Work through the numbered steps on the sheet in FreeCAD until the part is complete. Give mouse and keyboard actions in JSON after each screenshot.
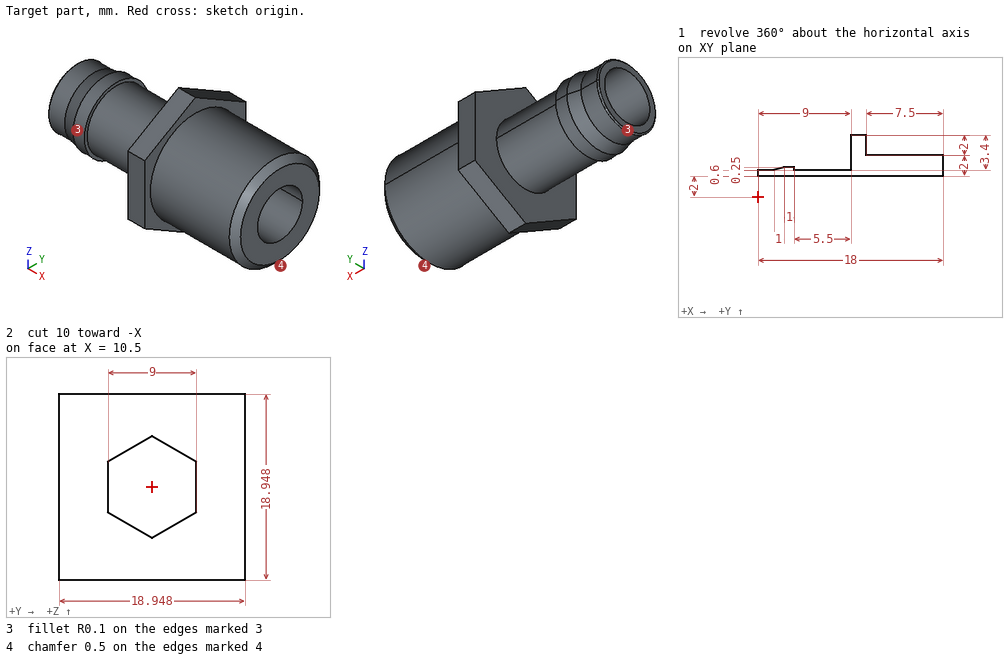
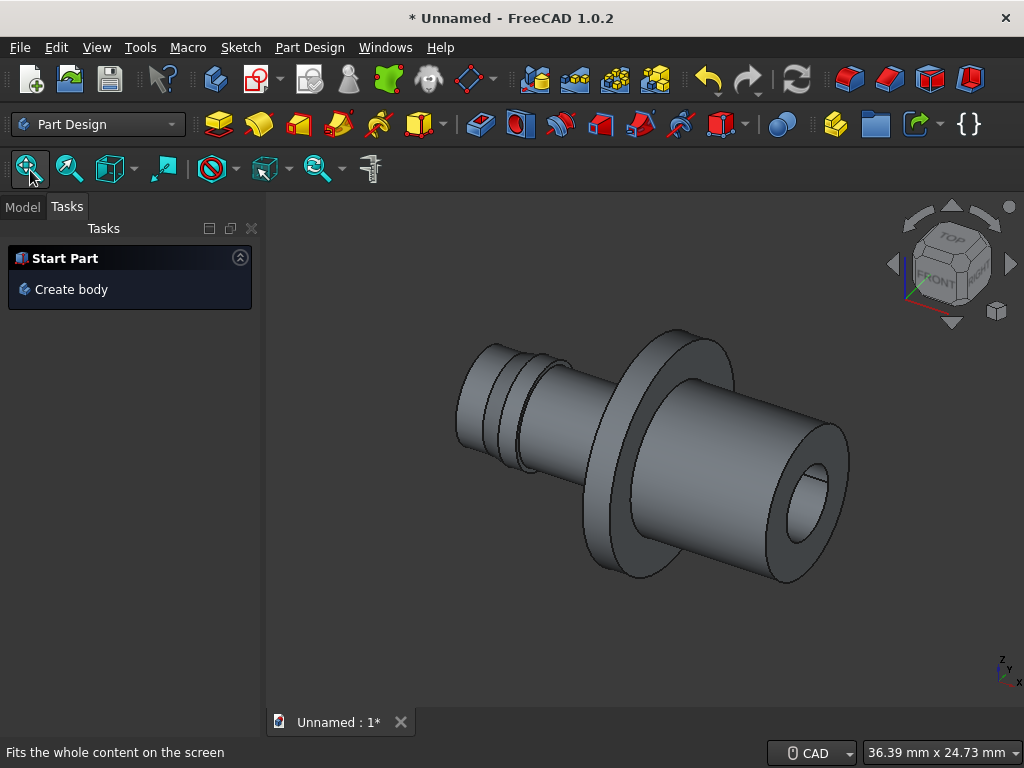
{"action": "left_click", "coordinate": [672, 370]}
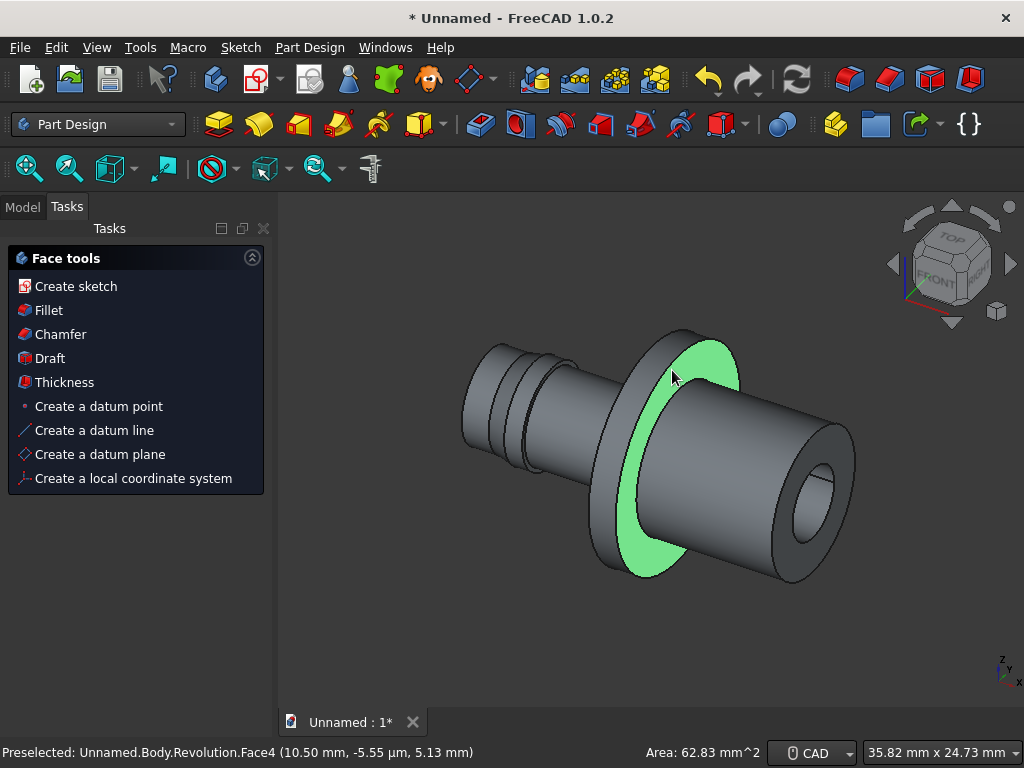
{"action": "left_click", "coordinate": [256, 80]}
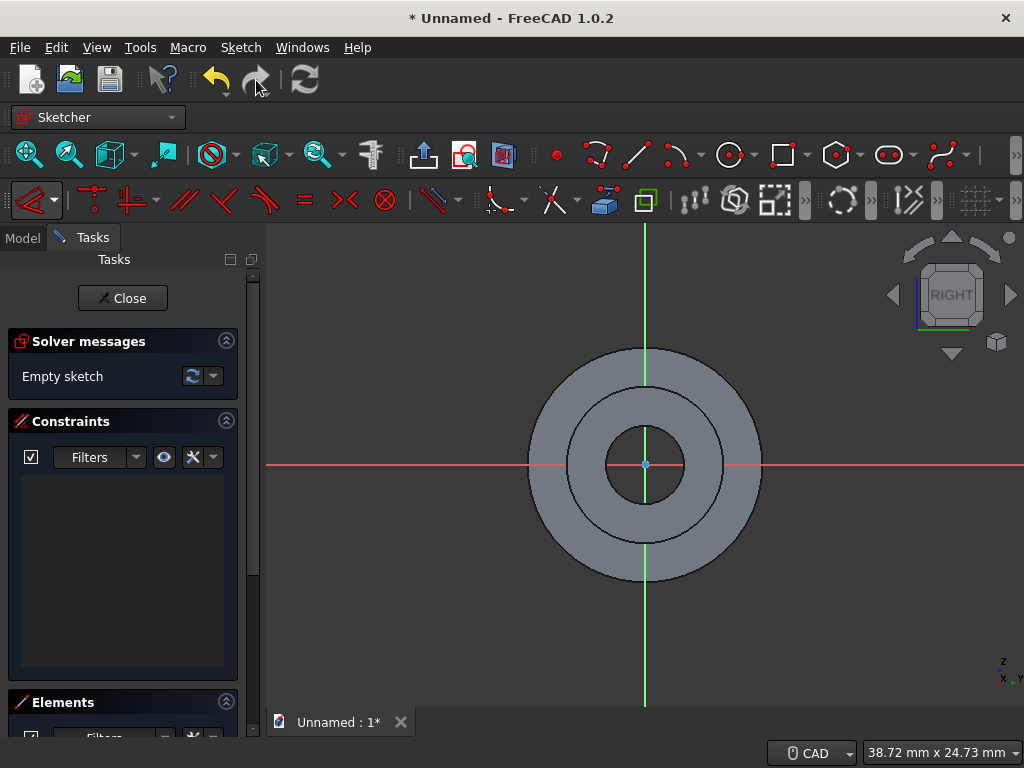
{"action": "left_click", "coordinate": [504, 156]}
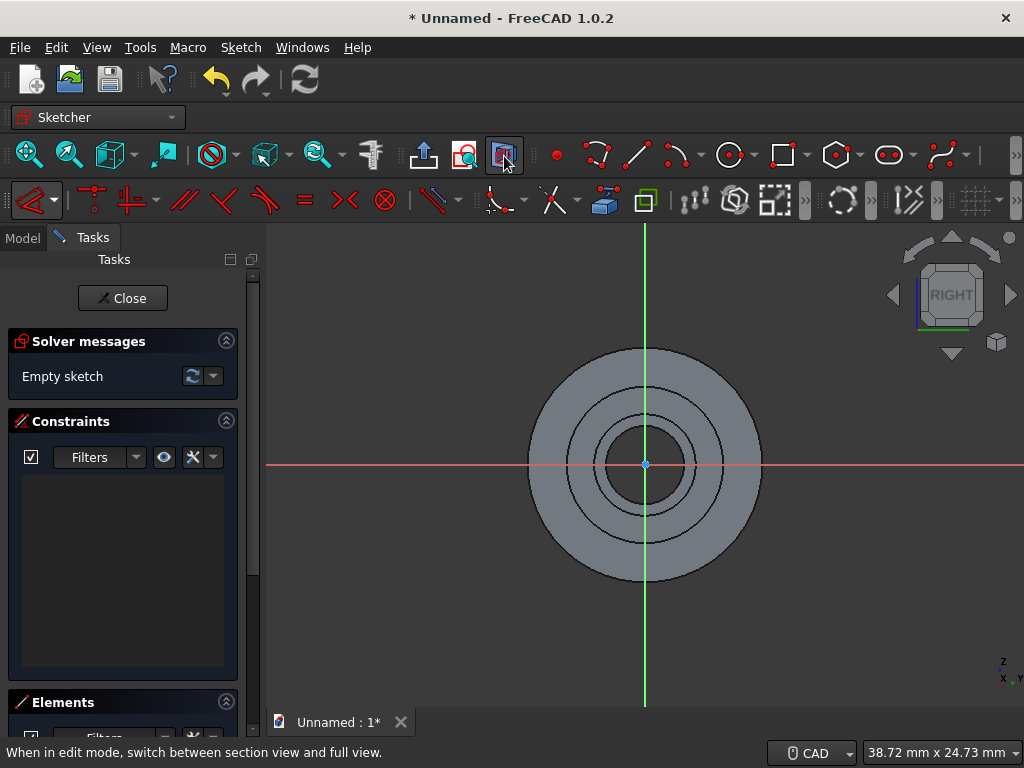
{"action": "left_click", "coordinate": [810, 156]}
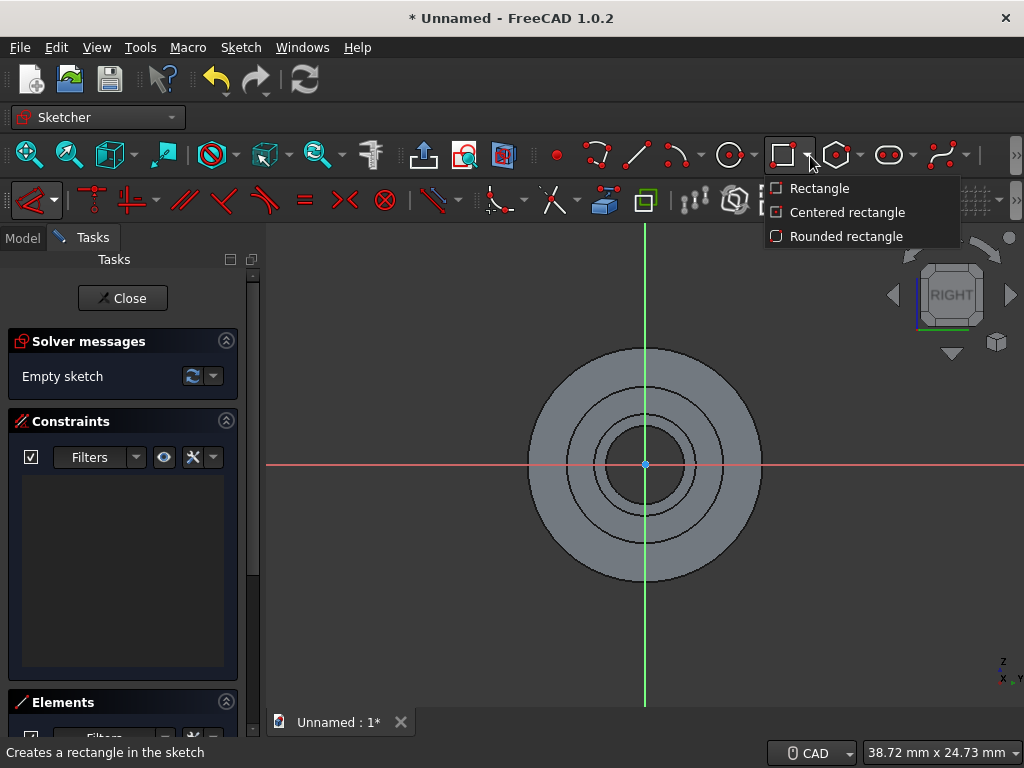
{"action": "left_click", "coordinate": [862, 212]}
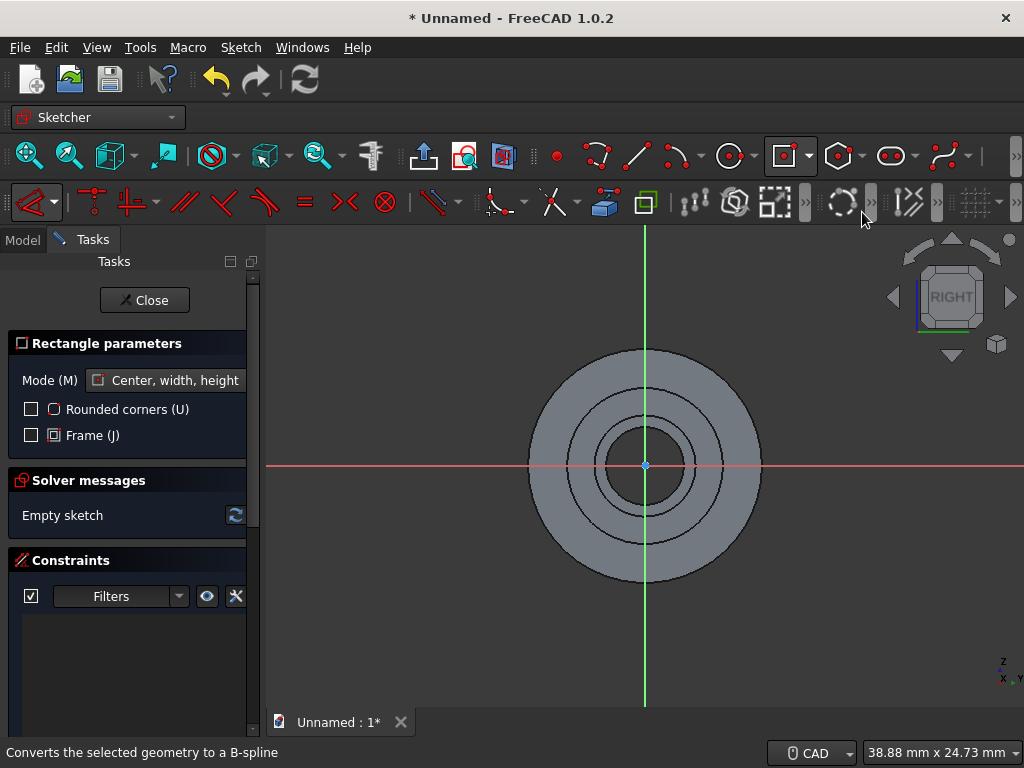
{"action": "left_click", "coordinate": [645, 466]}
{"action": "mouse_move", "coordinate": [830, 281]}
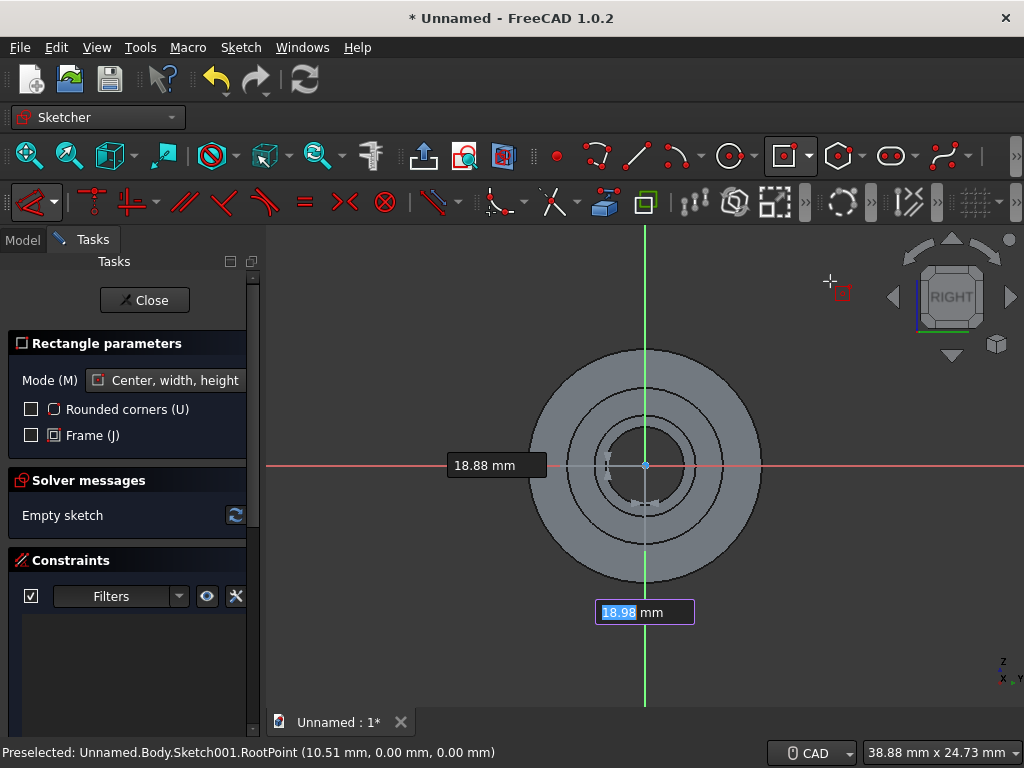
{"action": "type", "text": "18.948"}
{"action": "key", "text": "Tab"}
{"action": "type", "text": "18.948"}
{"action": "key", "text": "Return"}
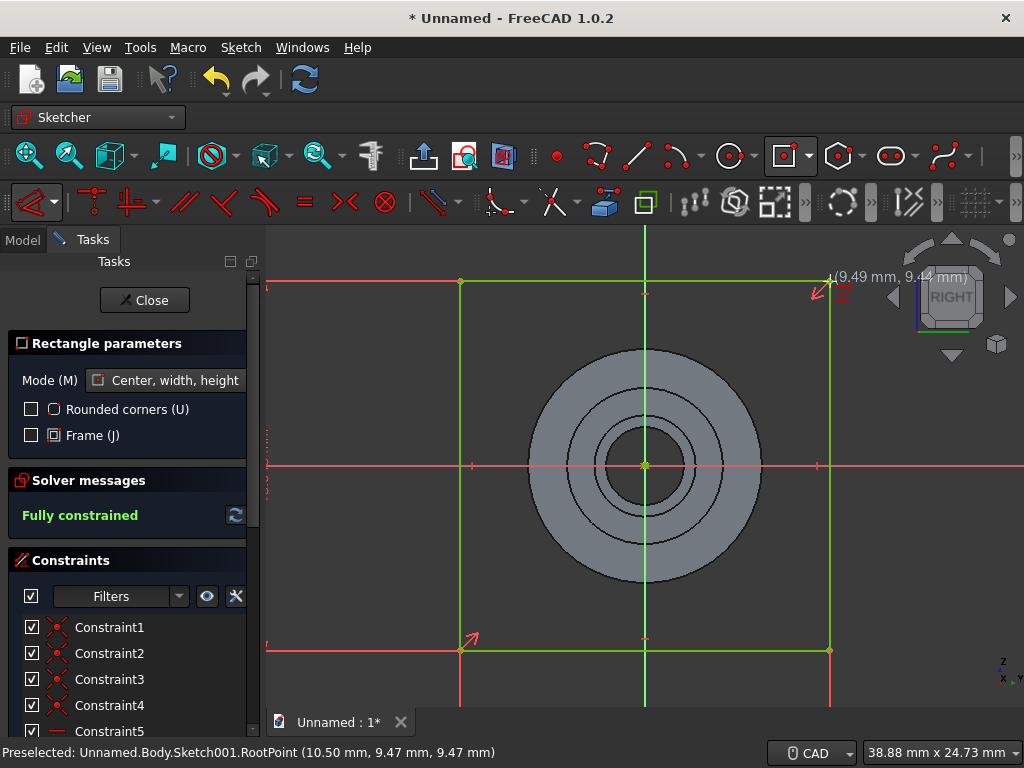
{"action": "key", "text": "g p 6"}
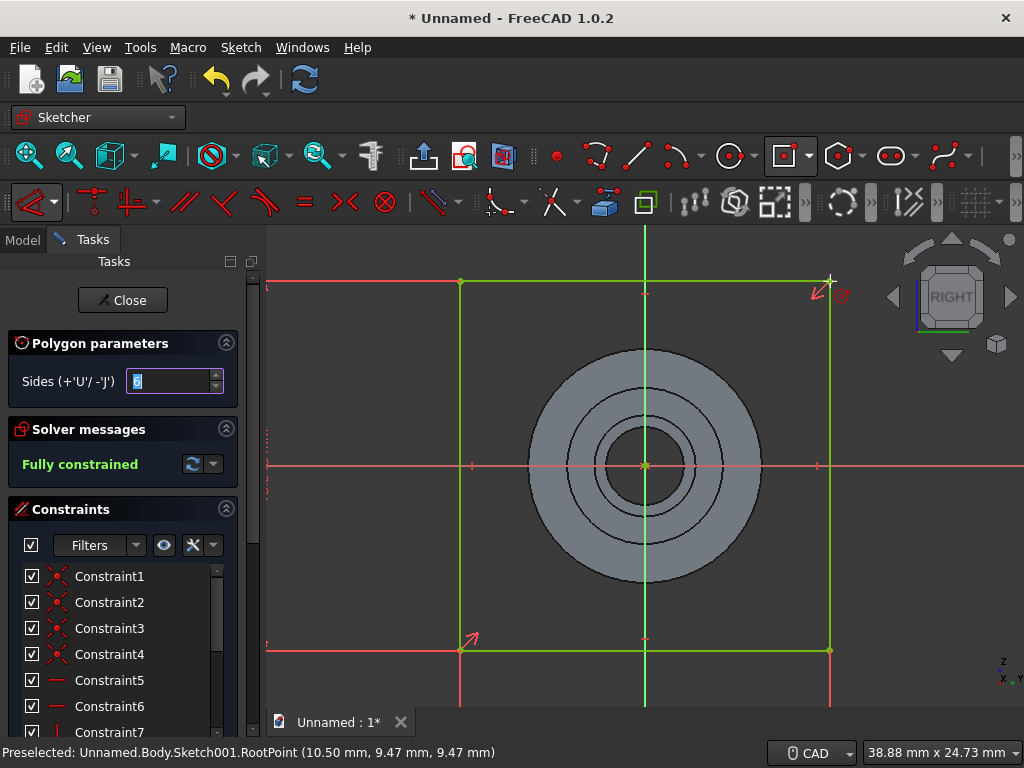
{"action": "left_click", "coordinate": [645, 466]}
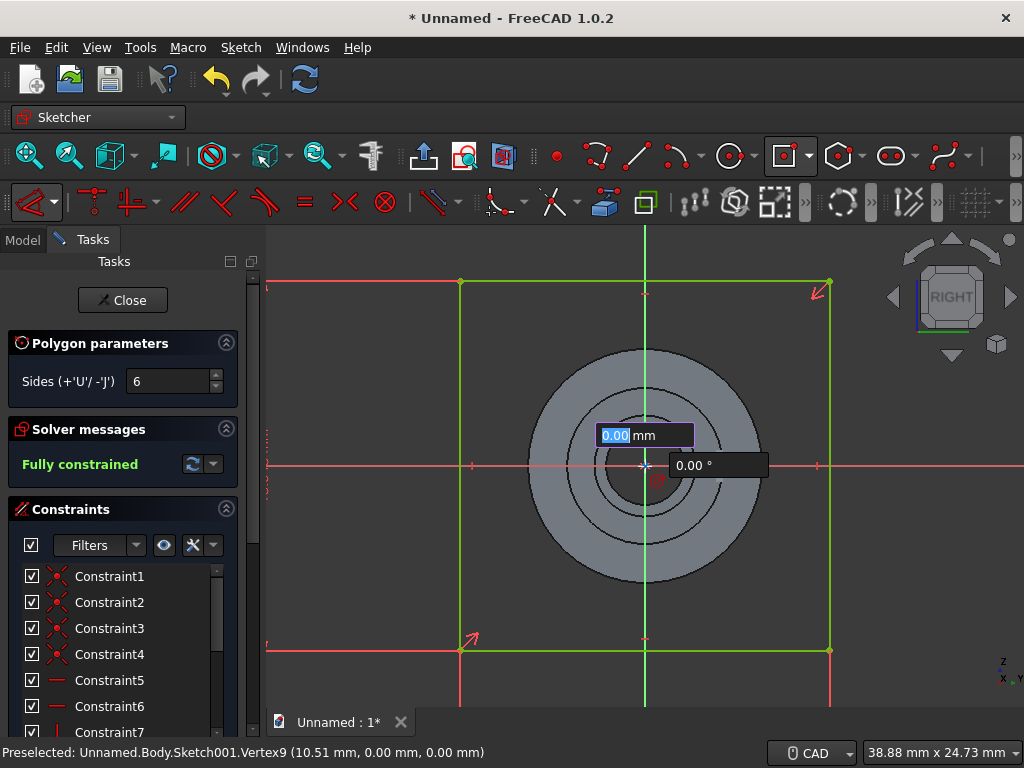
{"action": "left_click", "coordinate": [645, 567]}
{"action": "right_click", "coordinate": [645, 567]}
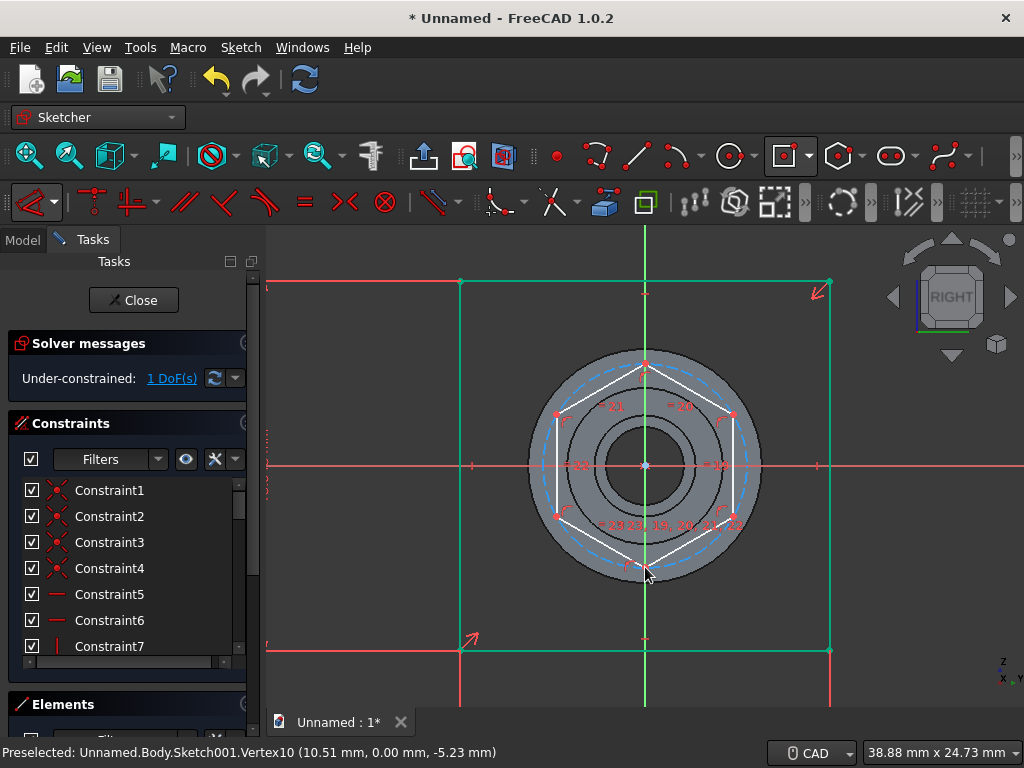
{"action": "left_click", "coordinate": [557, 415]}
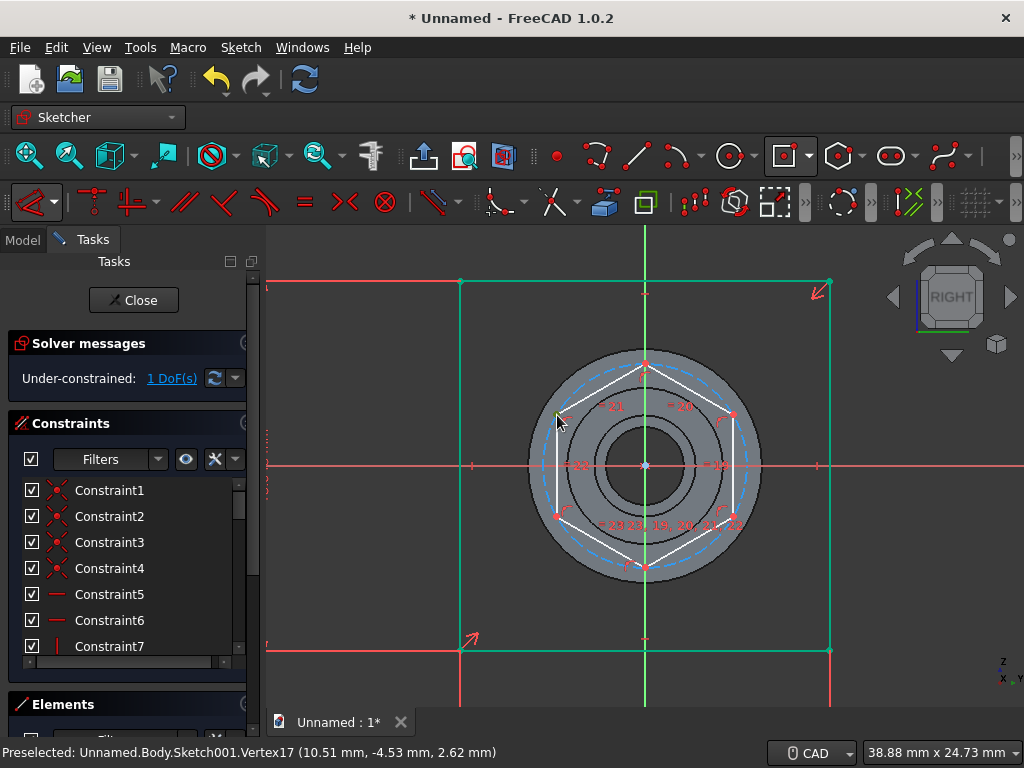
{"action": "left_click", "coordinate": [733, 517]}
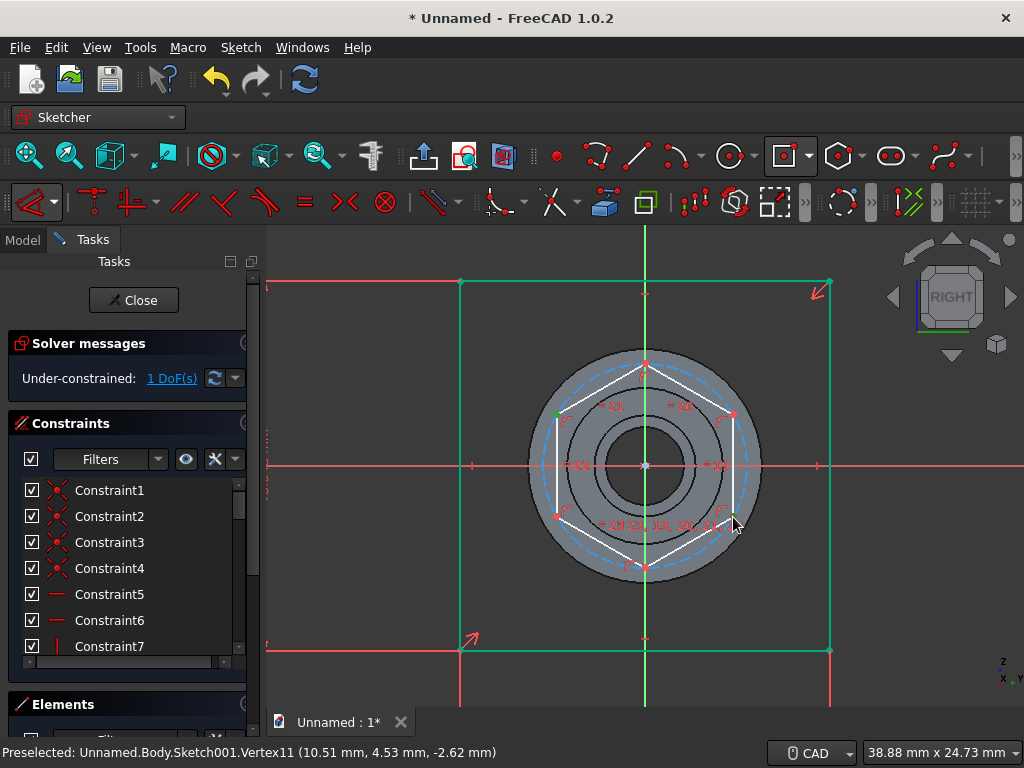
{"action": "key", "text": "l"}